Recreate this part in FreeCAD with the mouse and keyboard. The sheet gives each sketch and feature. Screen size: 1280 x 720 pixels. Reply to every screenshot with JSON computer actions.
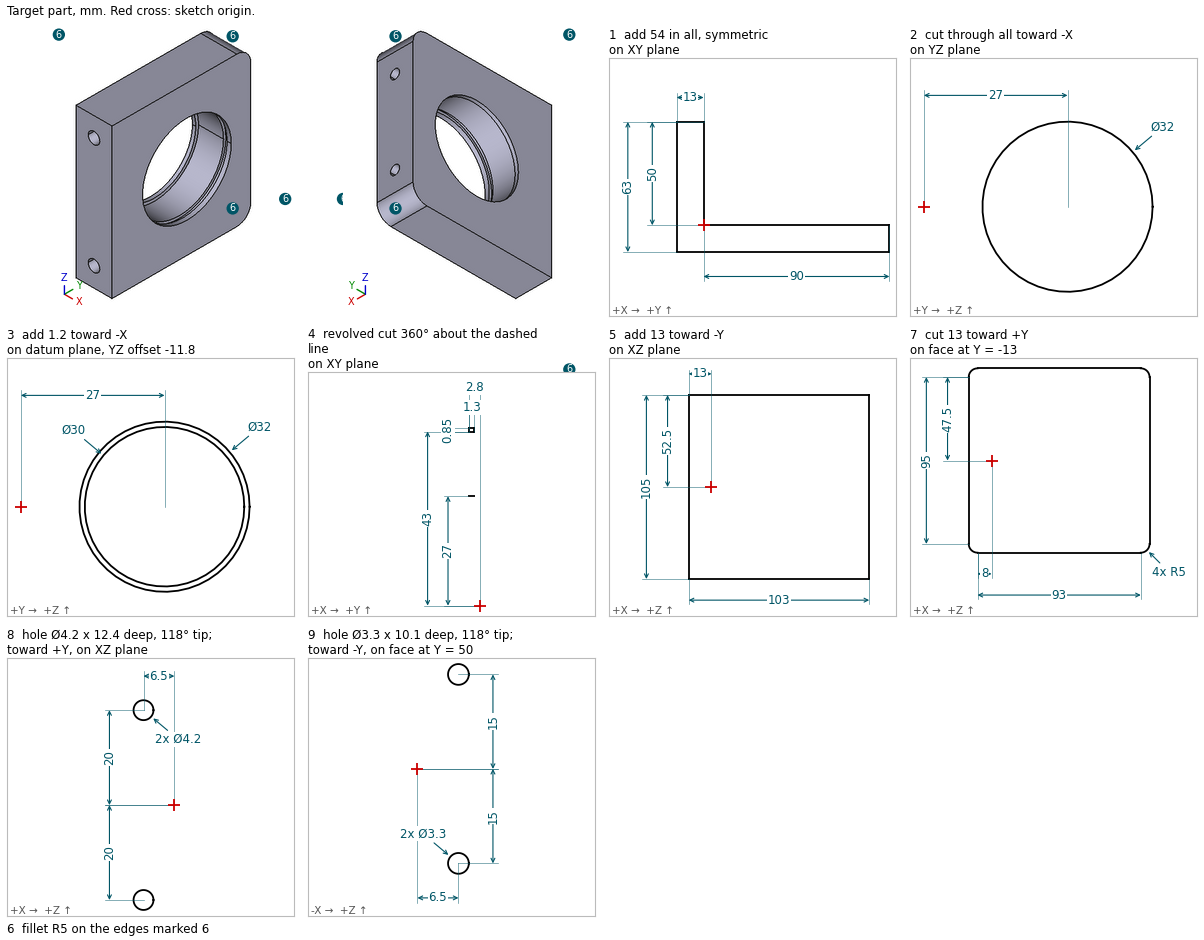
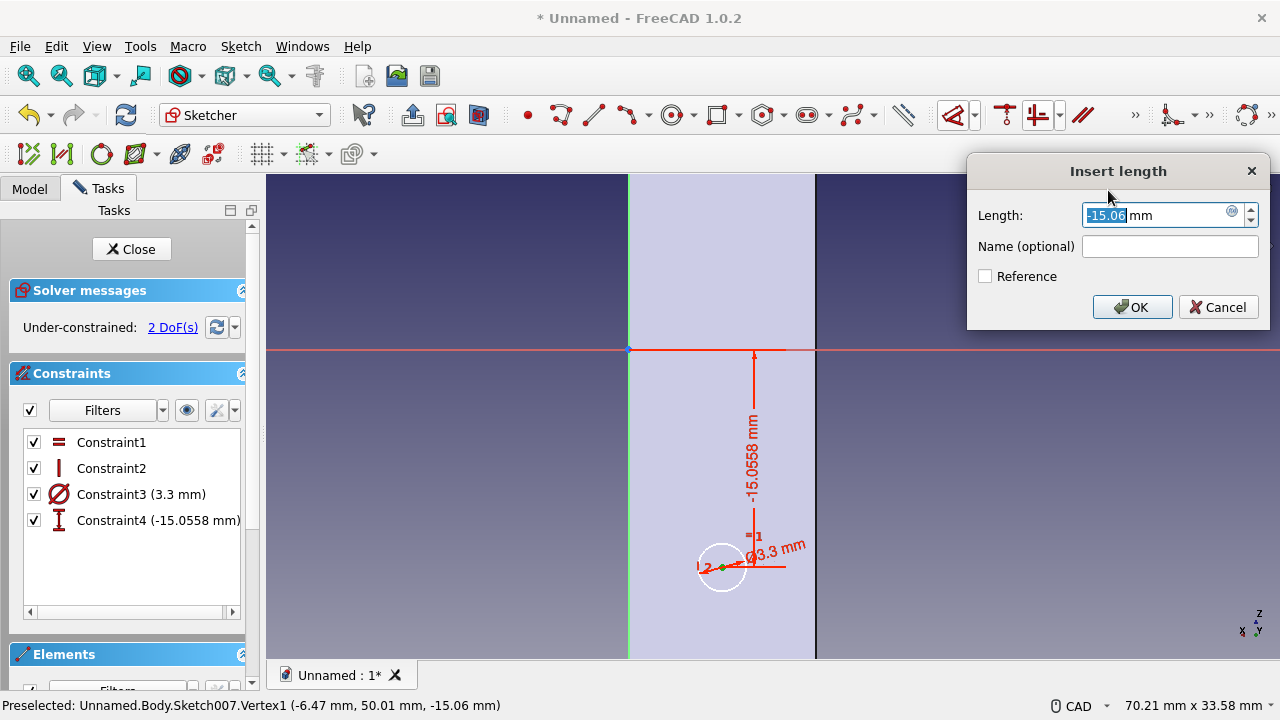
{"action": "type", "text": "-15"}
{"action": "key", "text": "Return"}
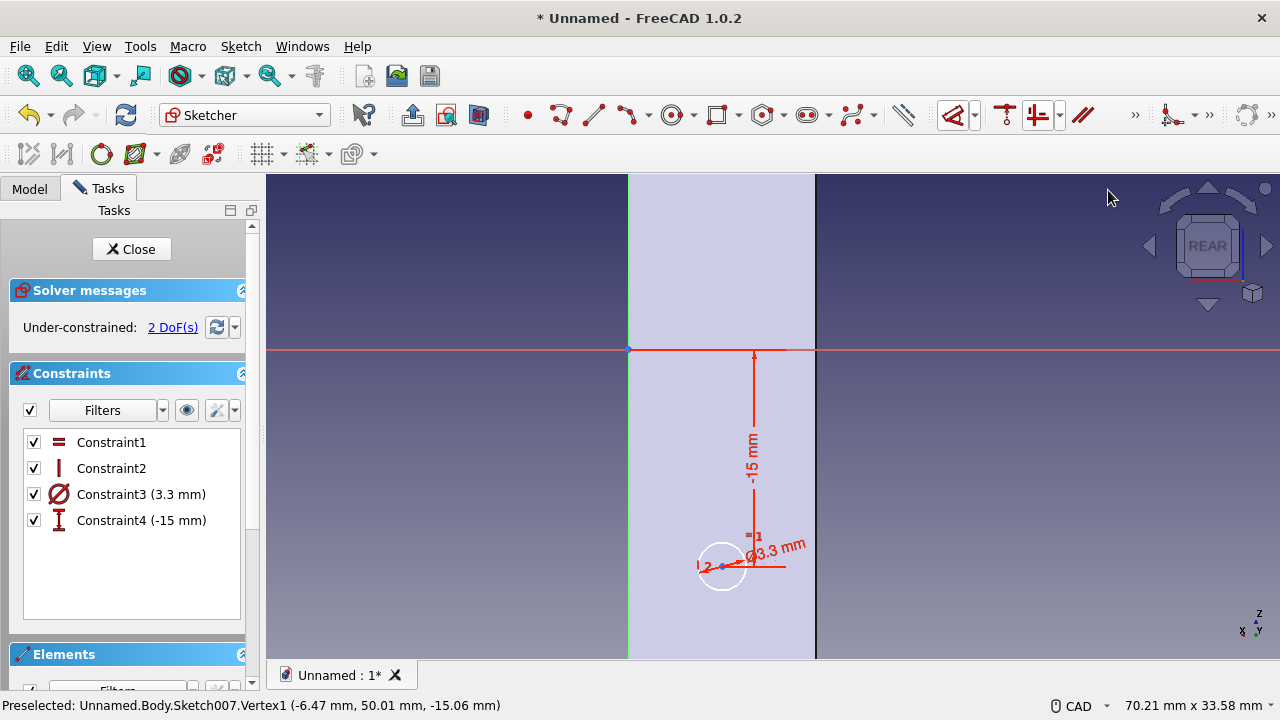
{"action": "scroll", "coordinate": [739, 552], "scroll_direction": "down", "scroll_amount": 2}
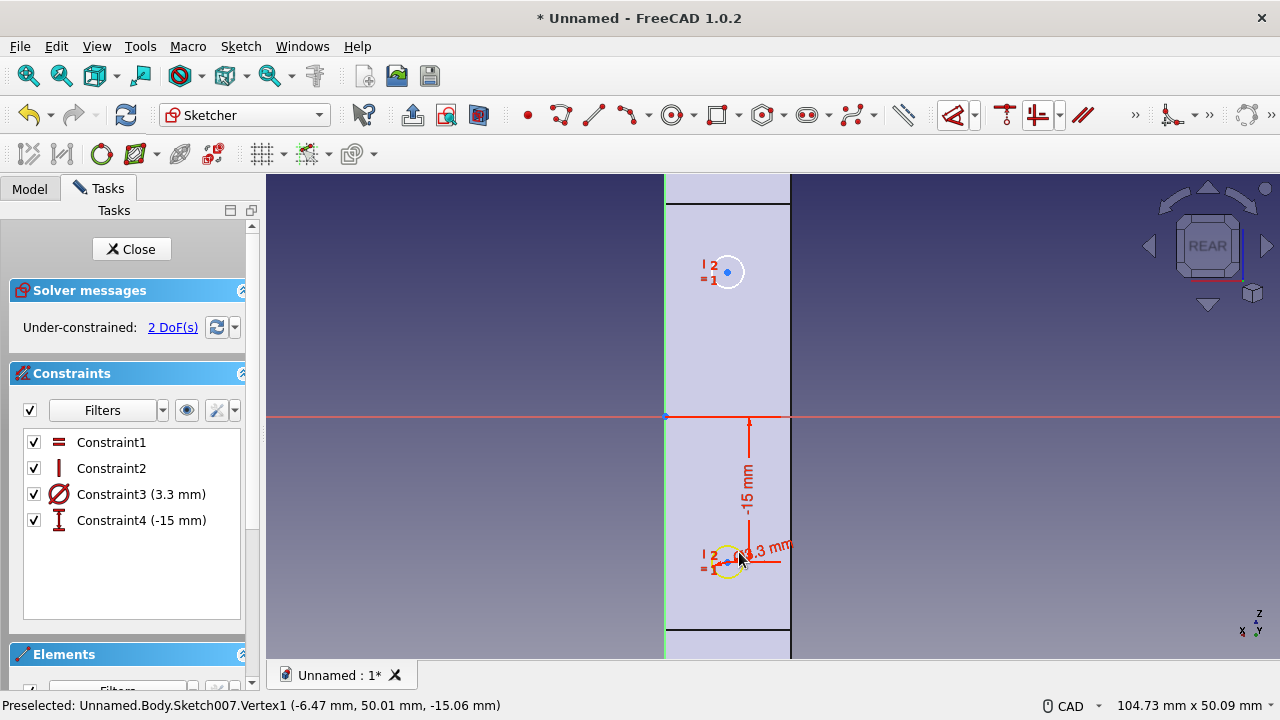
{"action": "left_click", "coordinate": [728, 272]}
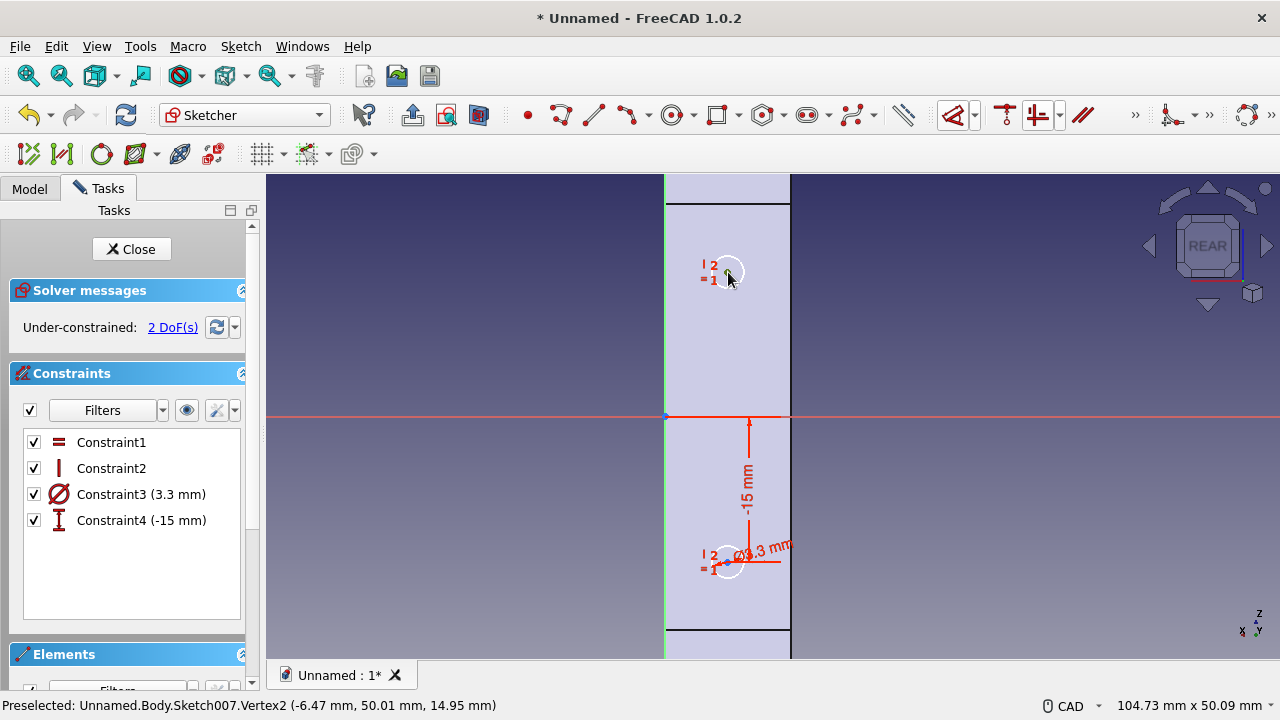
{"action": "key", "text": "i"}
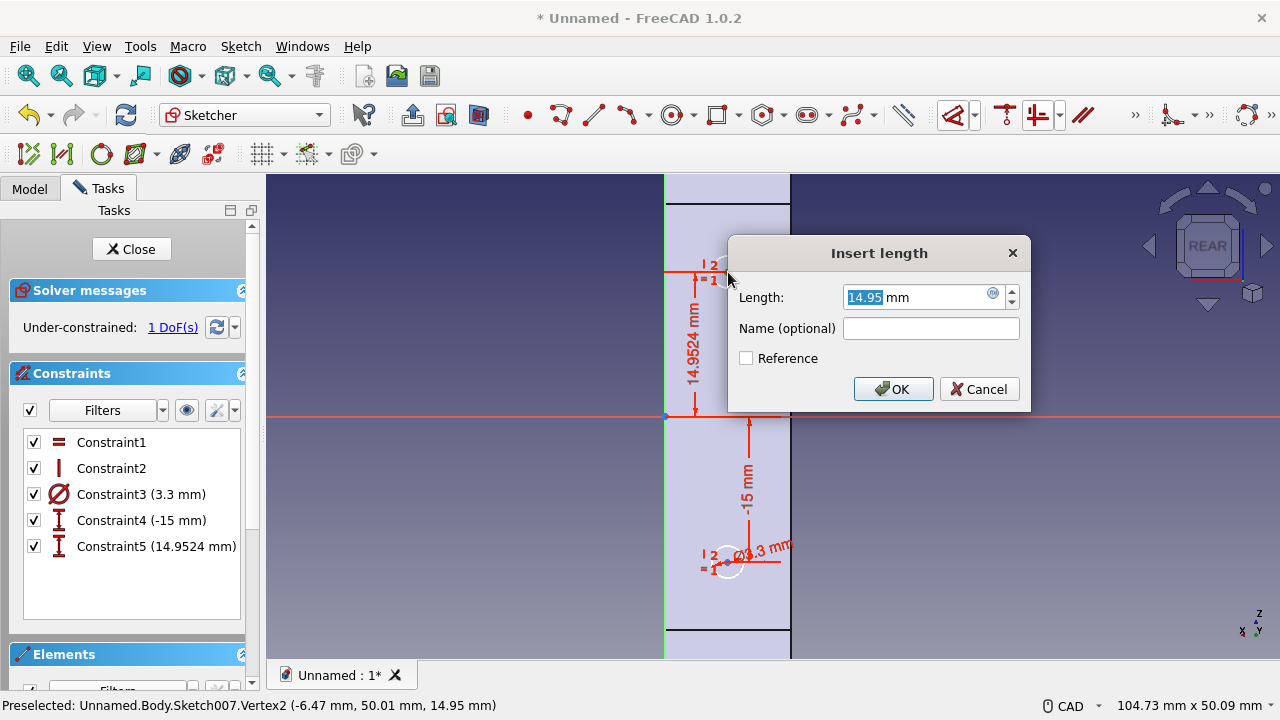
{"action": "type", "text": "15"}
{"action": "key", "text": "Return"}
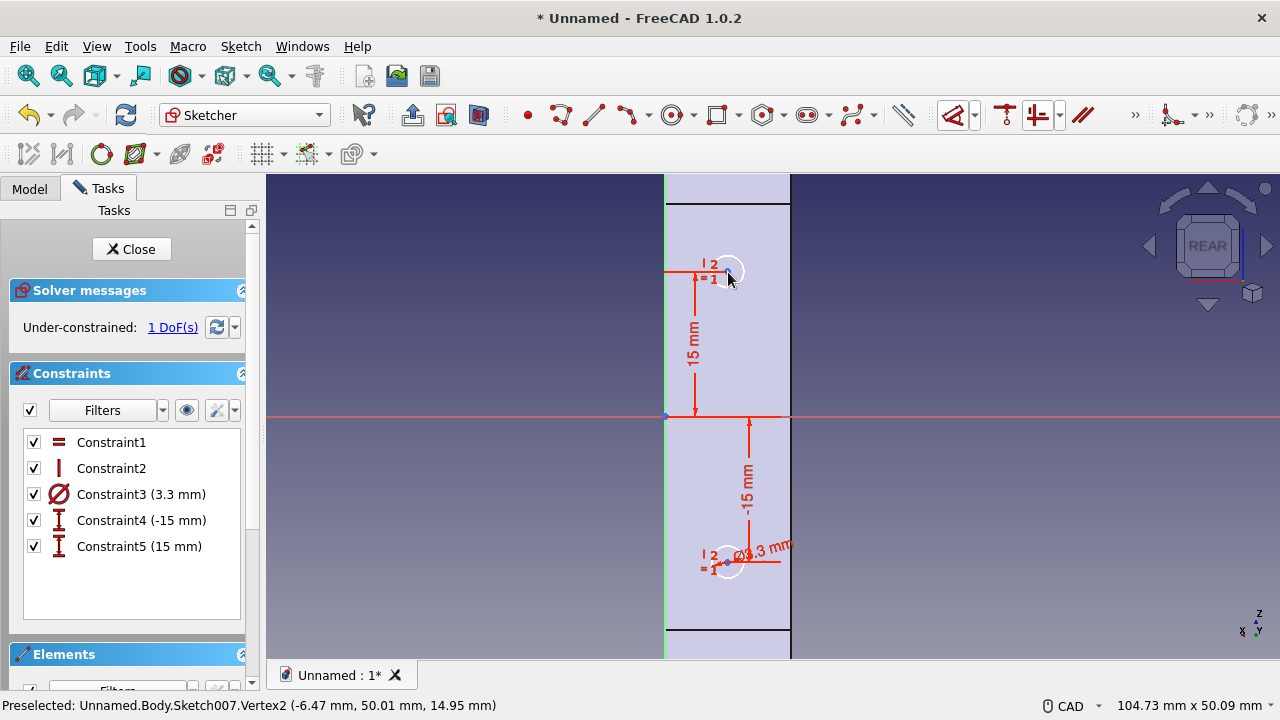
{"action": "left_click", "coordinate": [728, 562]}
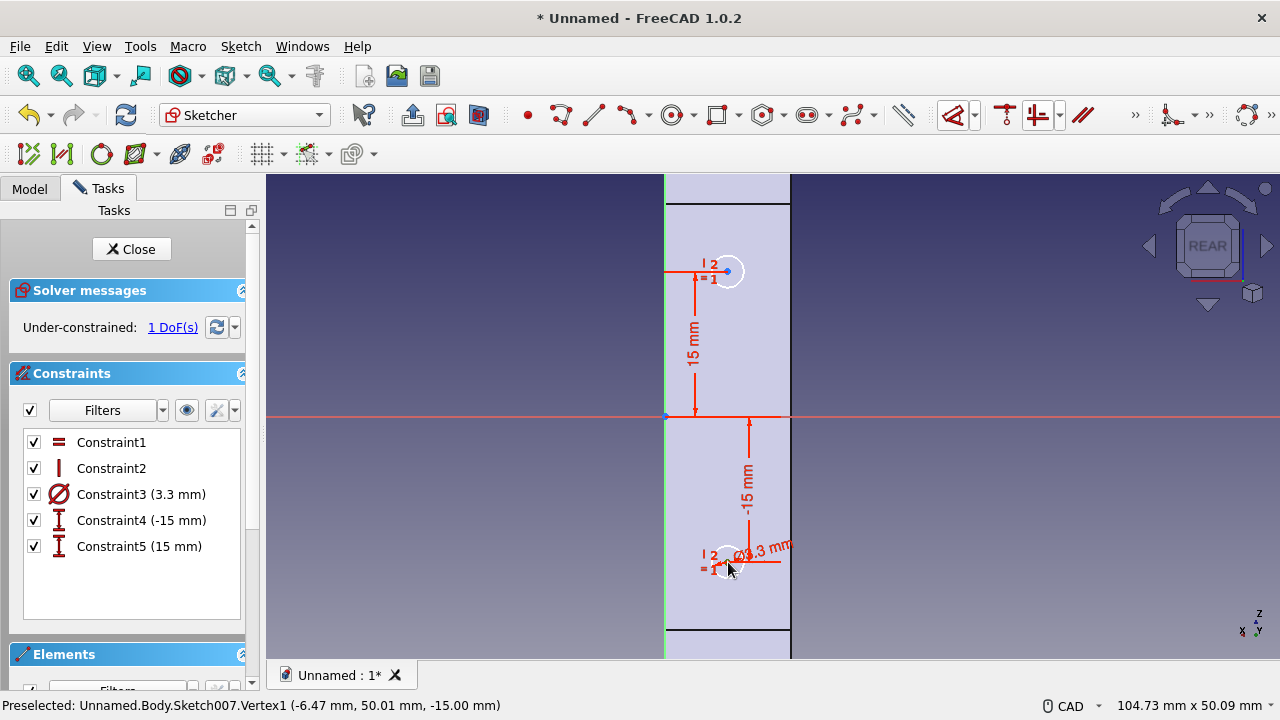
{"action": "left_click", "coordinate": [974, 116]}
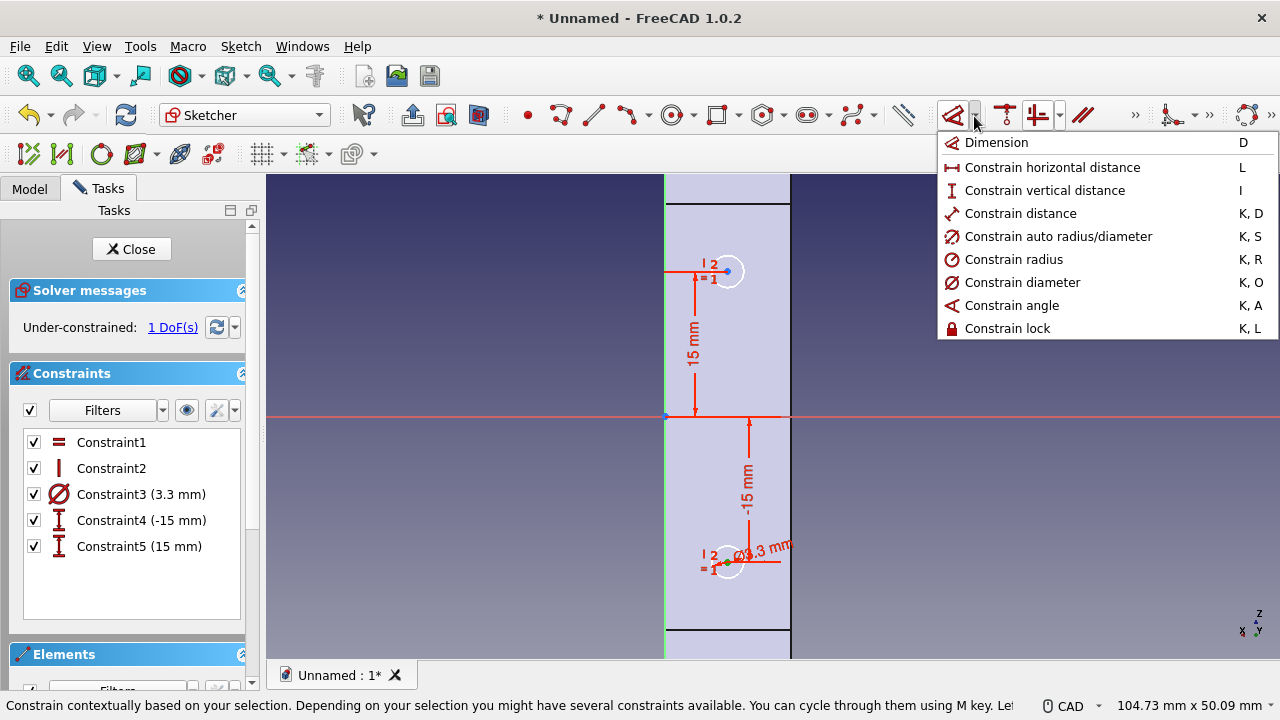
{"action": "left_click", "coordinate": [1108, 168]}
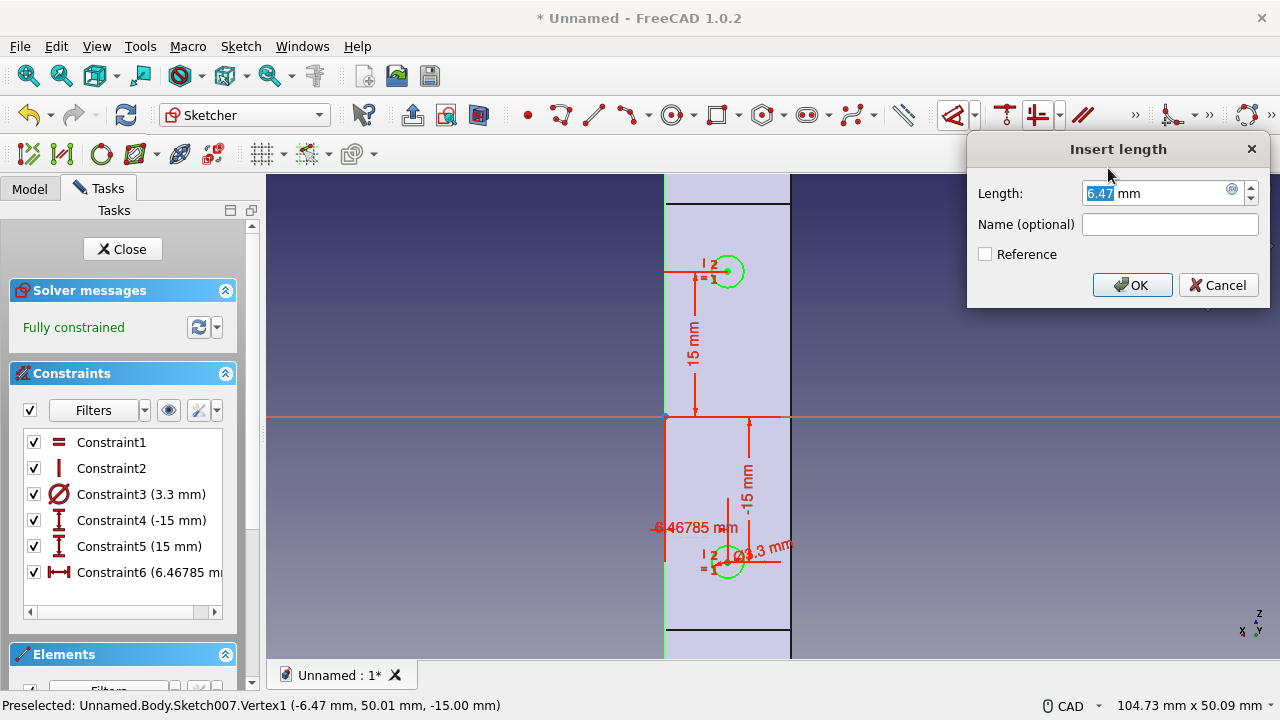
{"action": "type", "text": "6.5"}
{"action": "key", "text": "Return"}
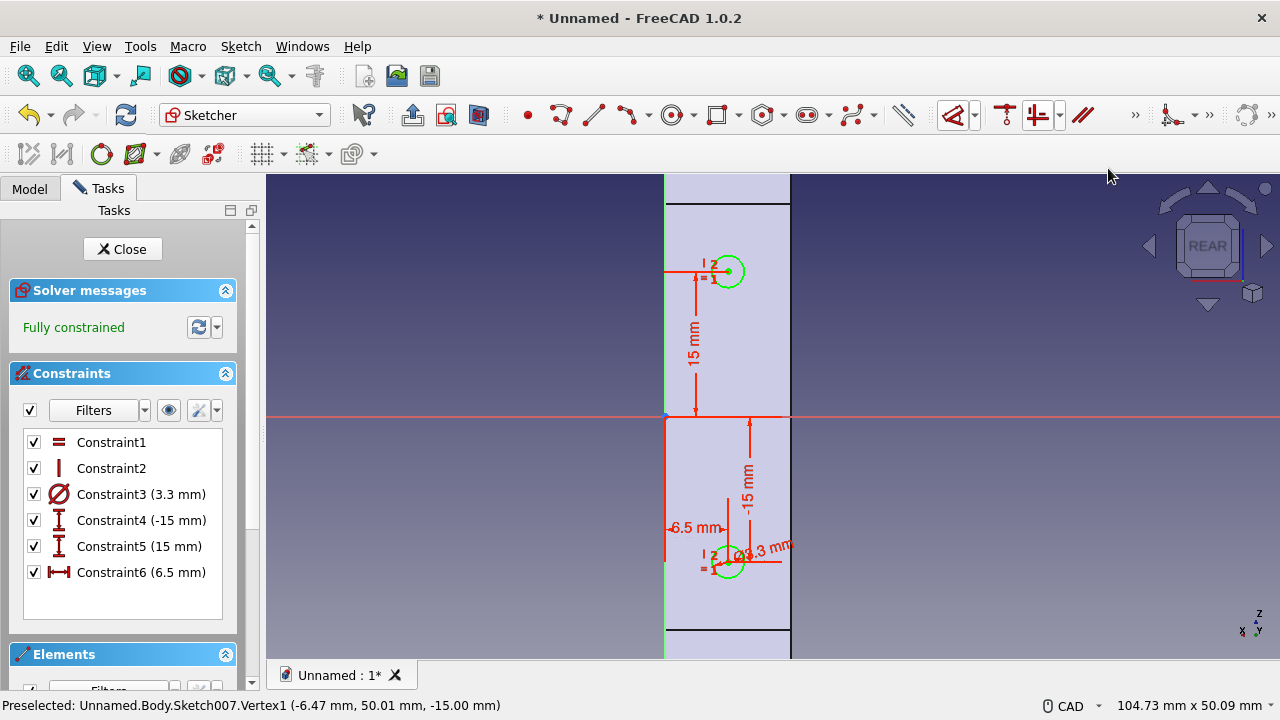
{"action": "left_click", "coordinate": [123, 249]}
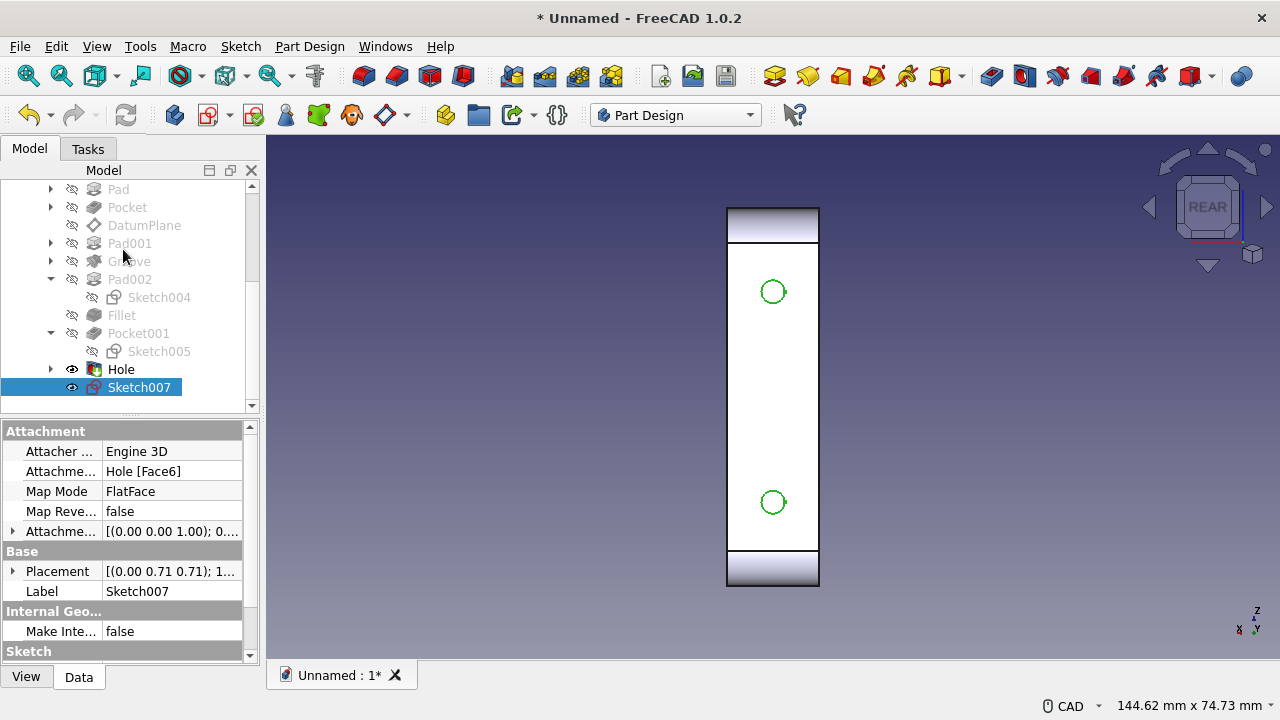
{"action": "left_click", "coordinate": [1025, 76]}